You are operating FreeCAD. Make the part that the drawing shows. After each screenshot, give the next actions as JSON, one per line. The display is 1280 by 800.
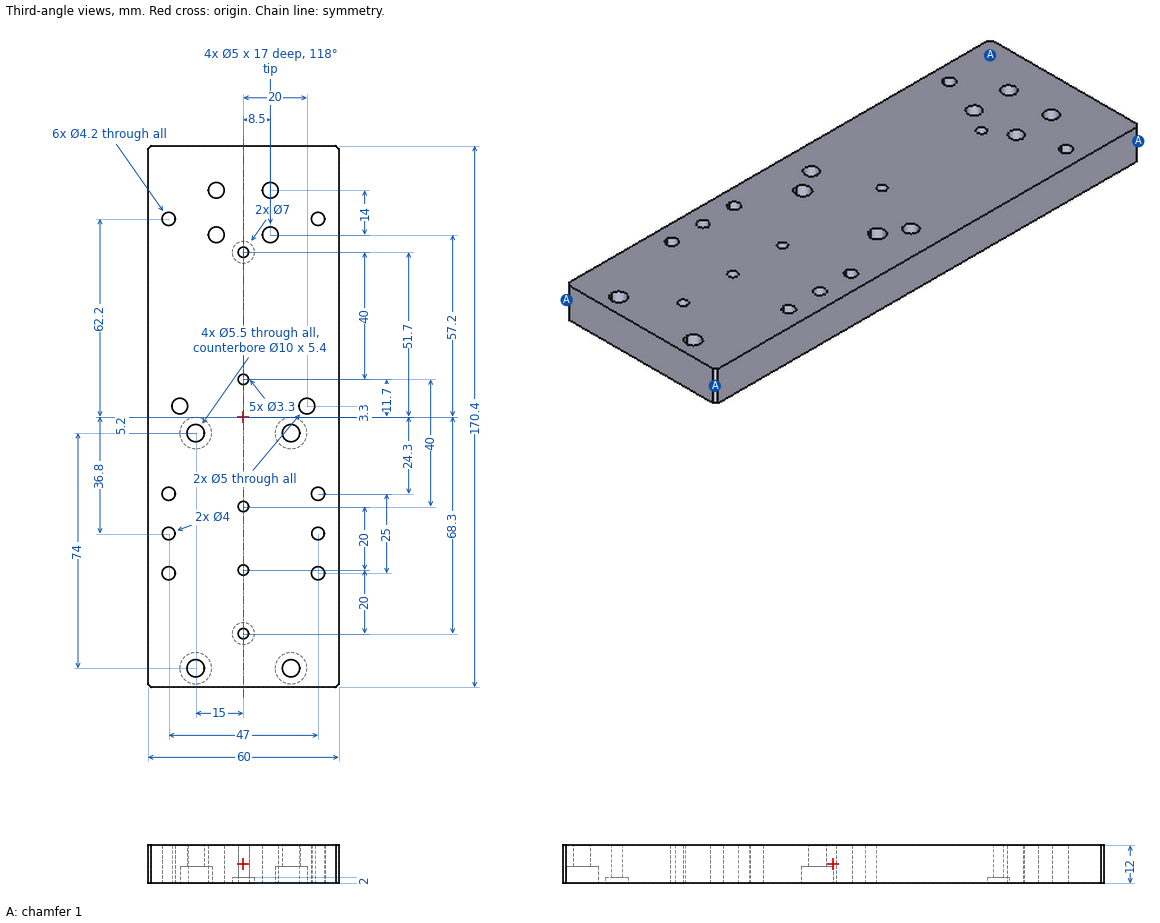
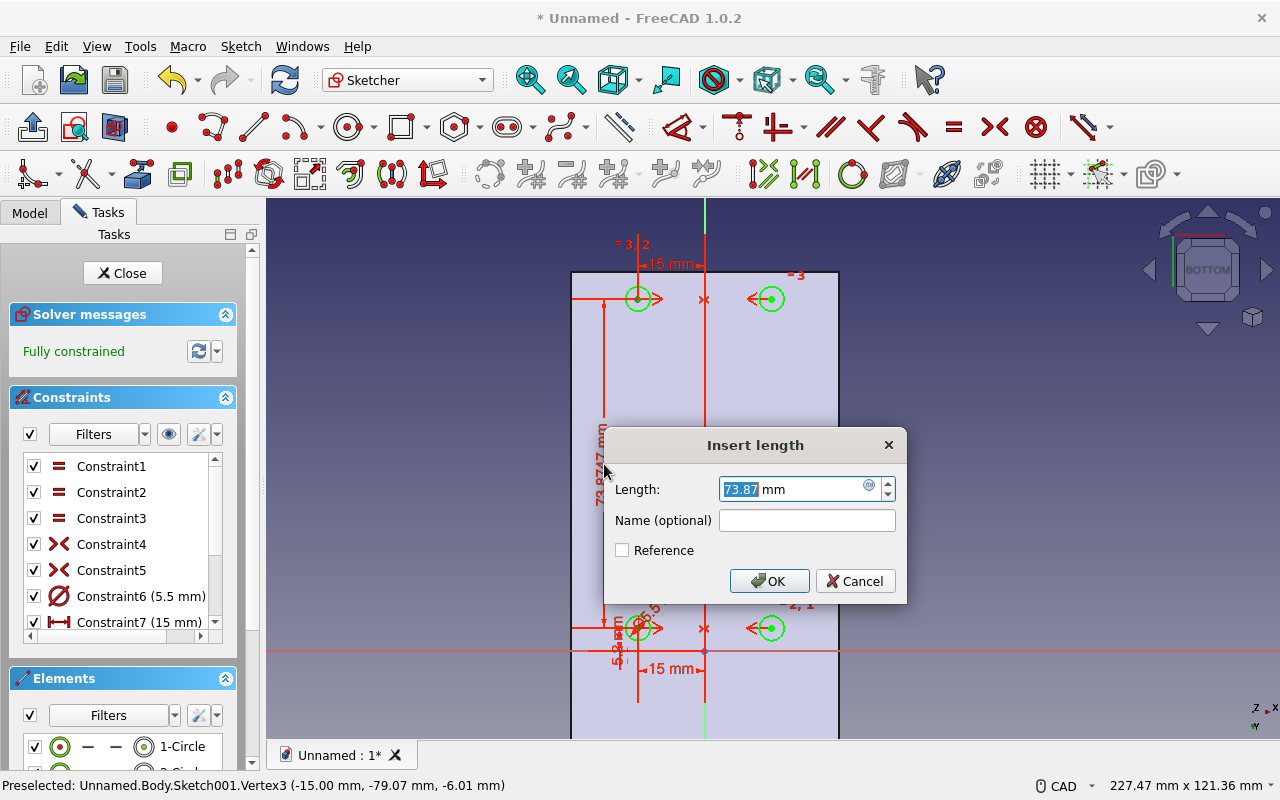
{"action": "type", "text": "74"}
{"action": "key", "text": "Return"}
{"action": "key", "text": "Escape"}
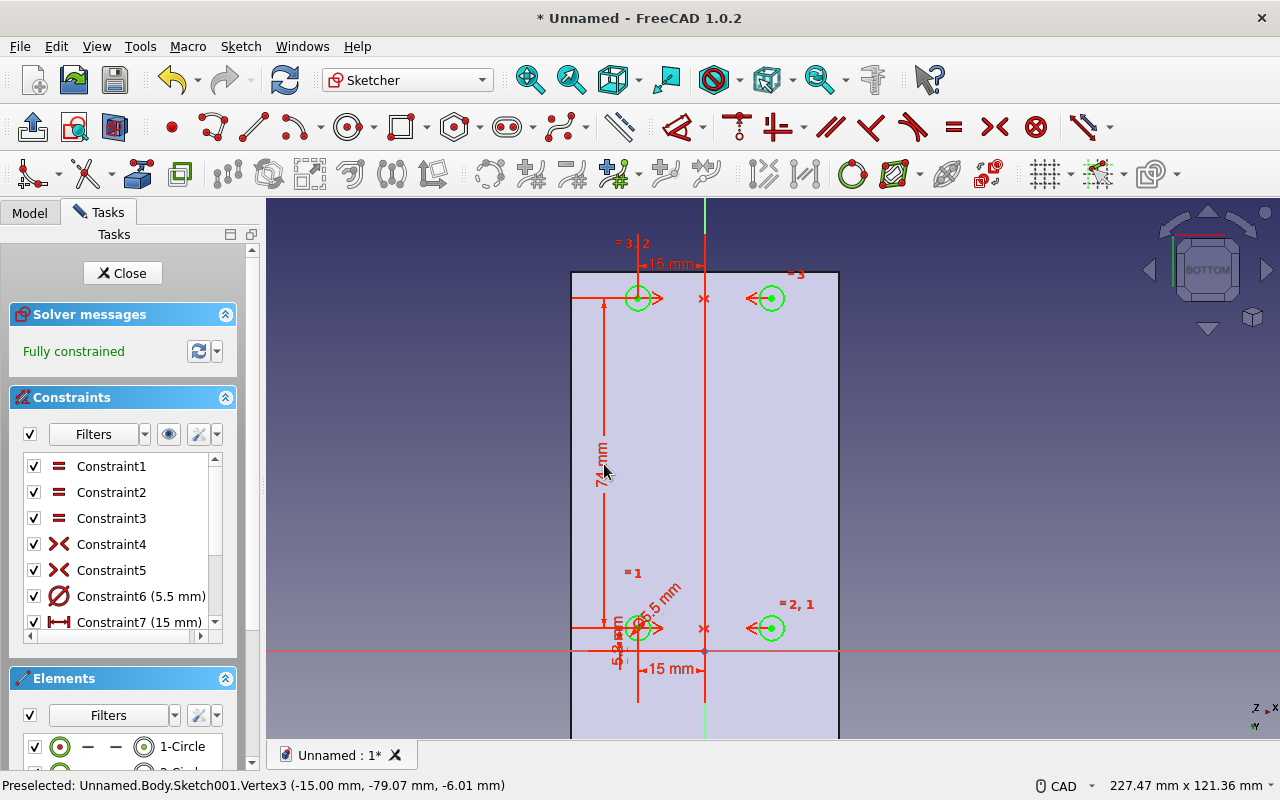
{"action": "left_click", "coordinate": [123, 273]}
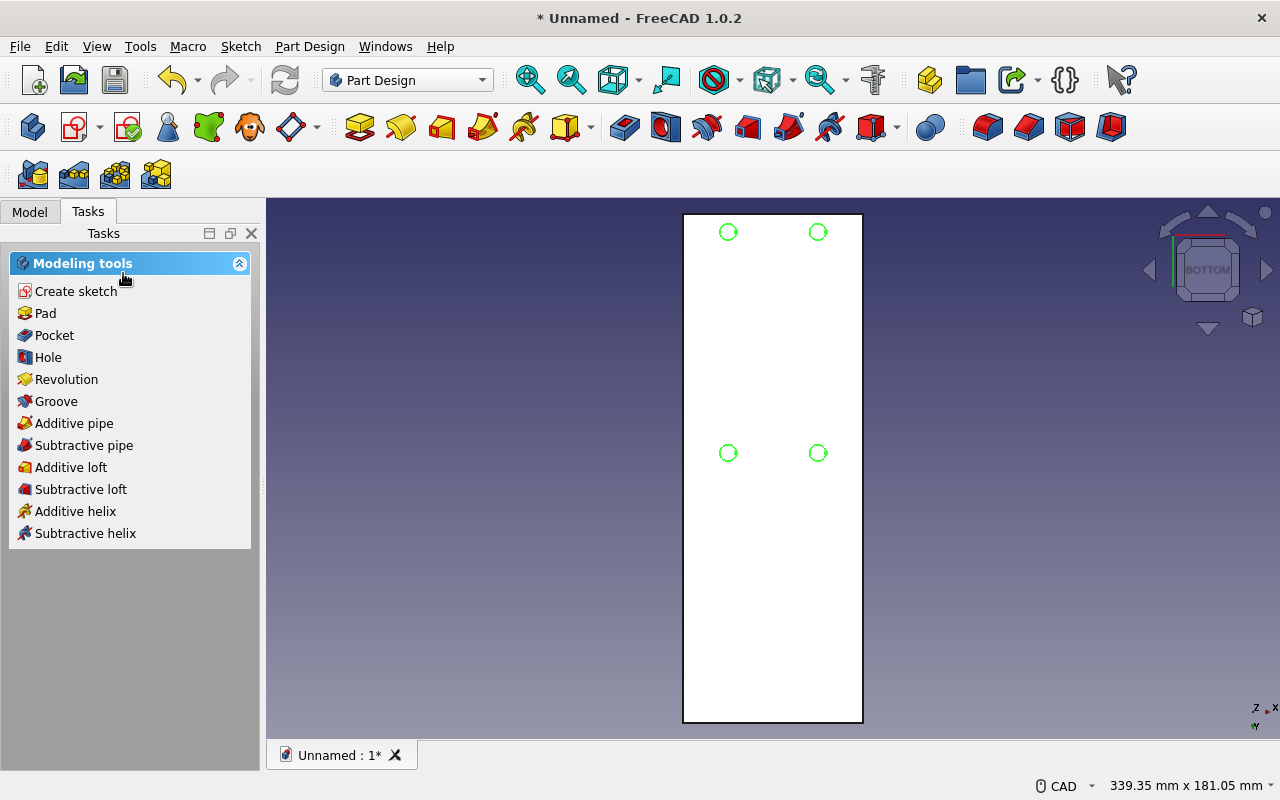
{"action": "left_click", "coordinate": [666, 128]}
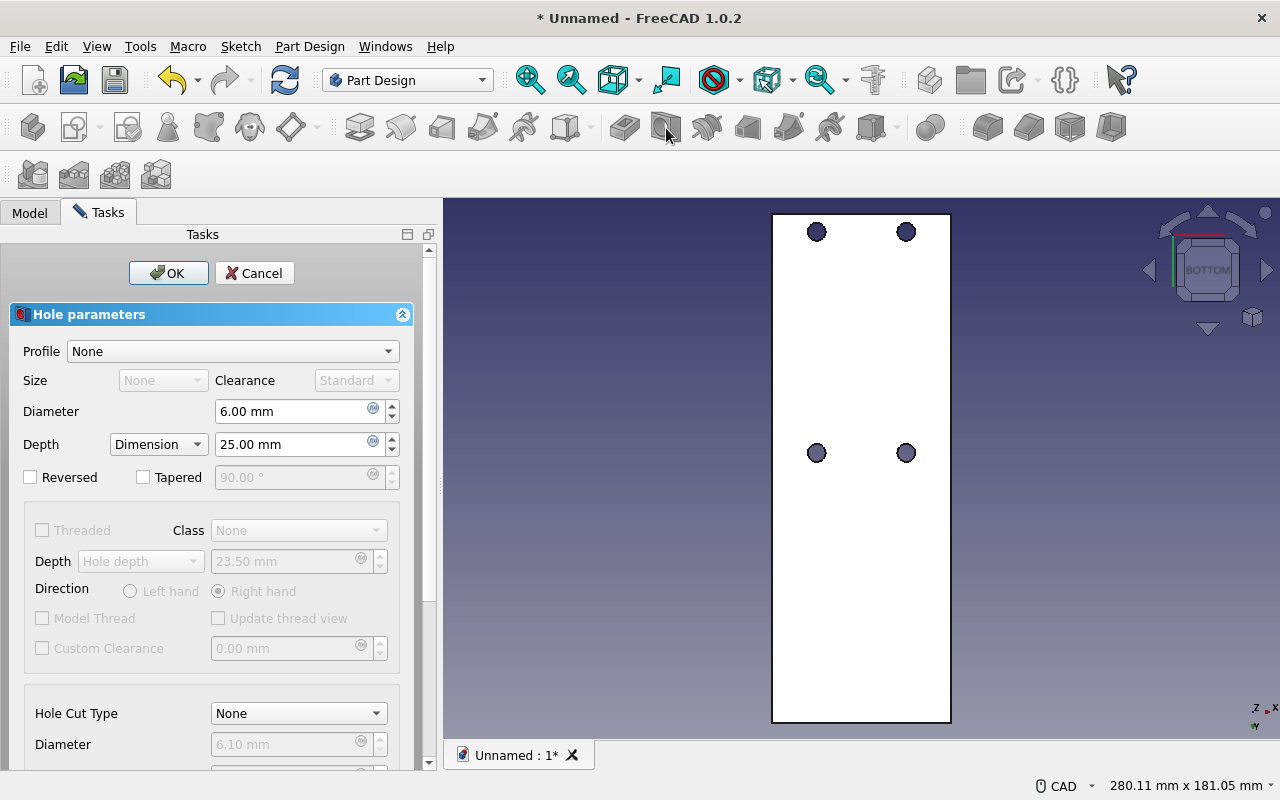
{"action": "triple_click", "coordinate": [300, 412]}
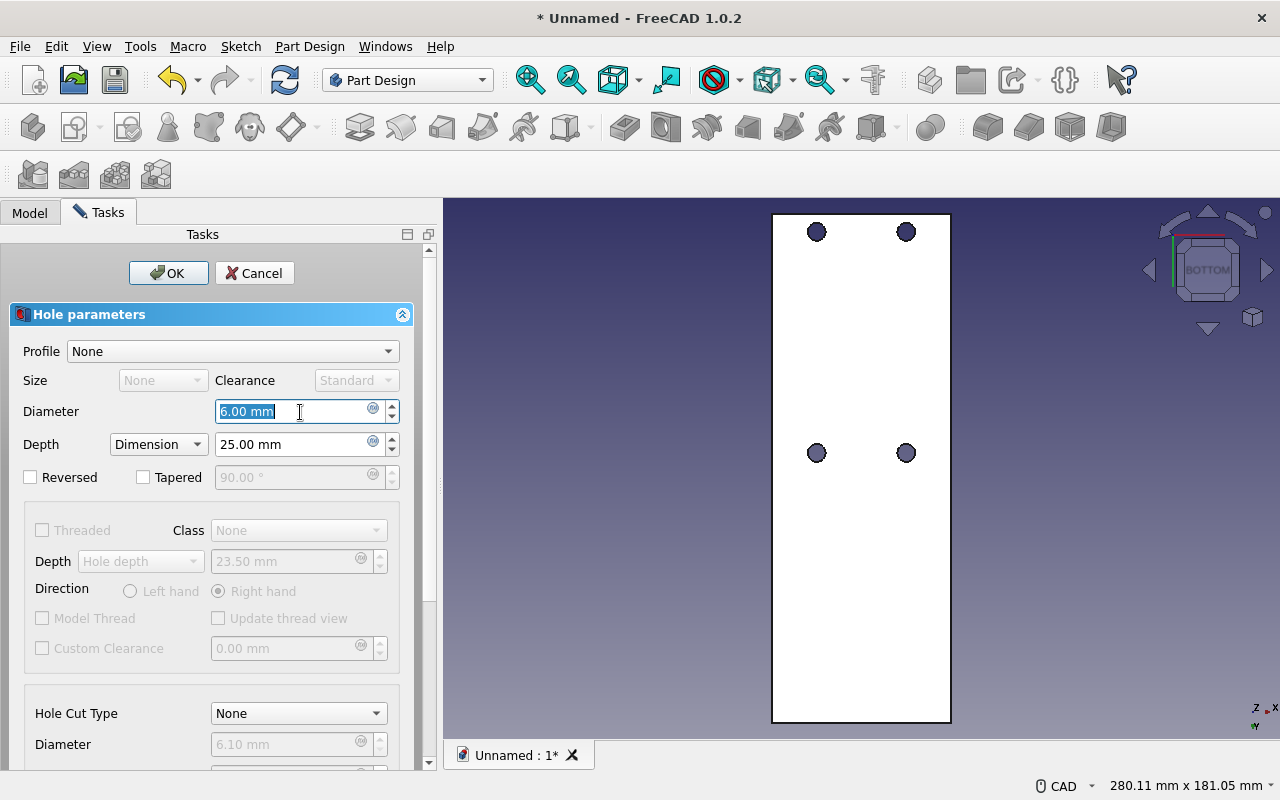
{"action": "type", "text": "5.5"}
{"action": "key", "text": "Tab"}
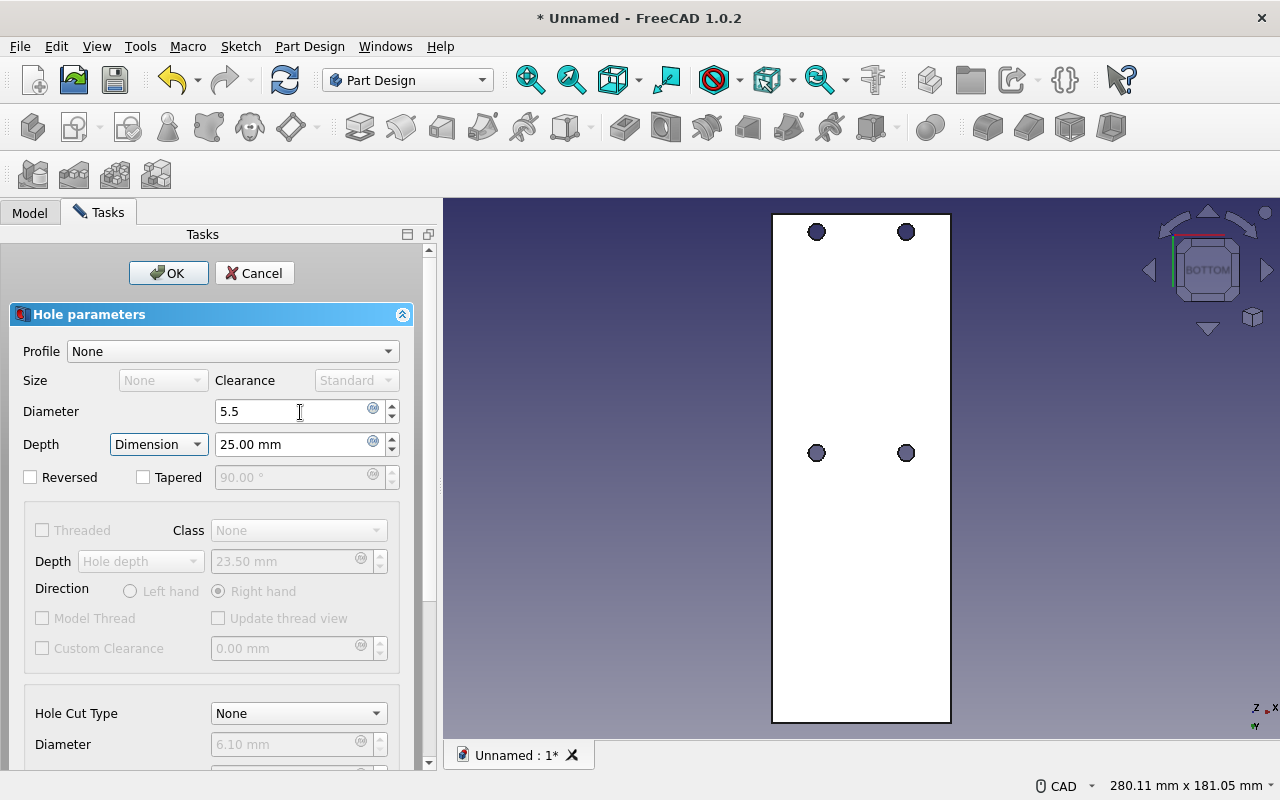
{"action": "left_click", "coordinate": [160, 444]}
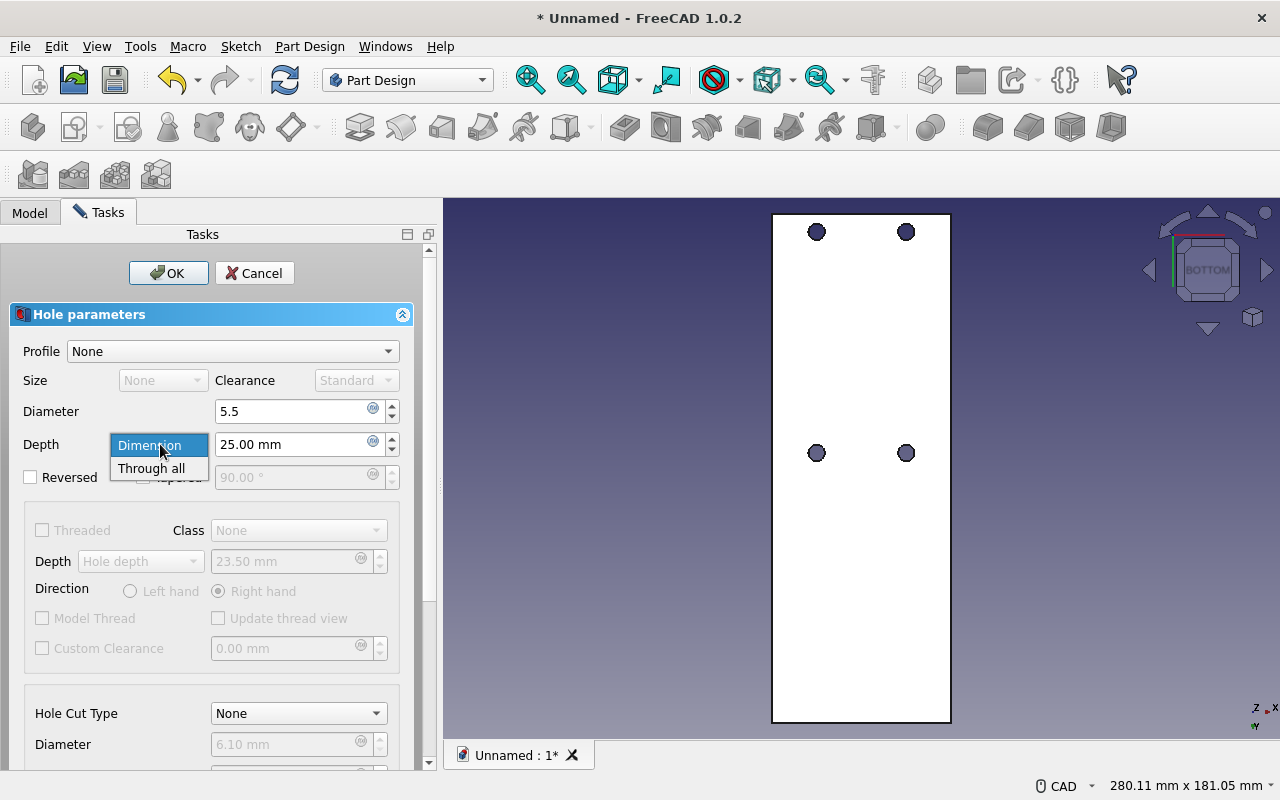
{"action": "left_click", "coordinate": [158, 468]}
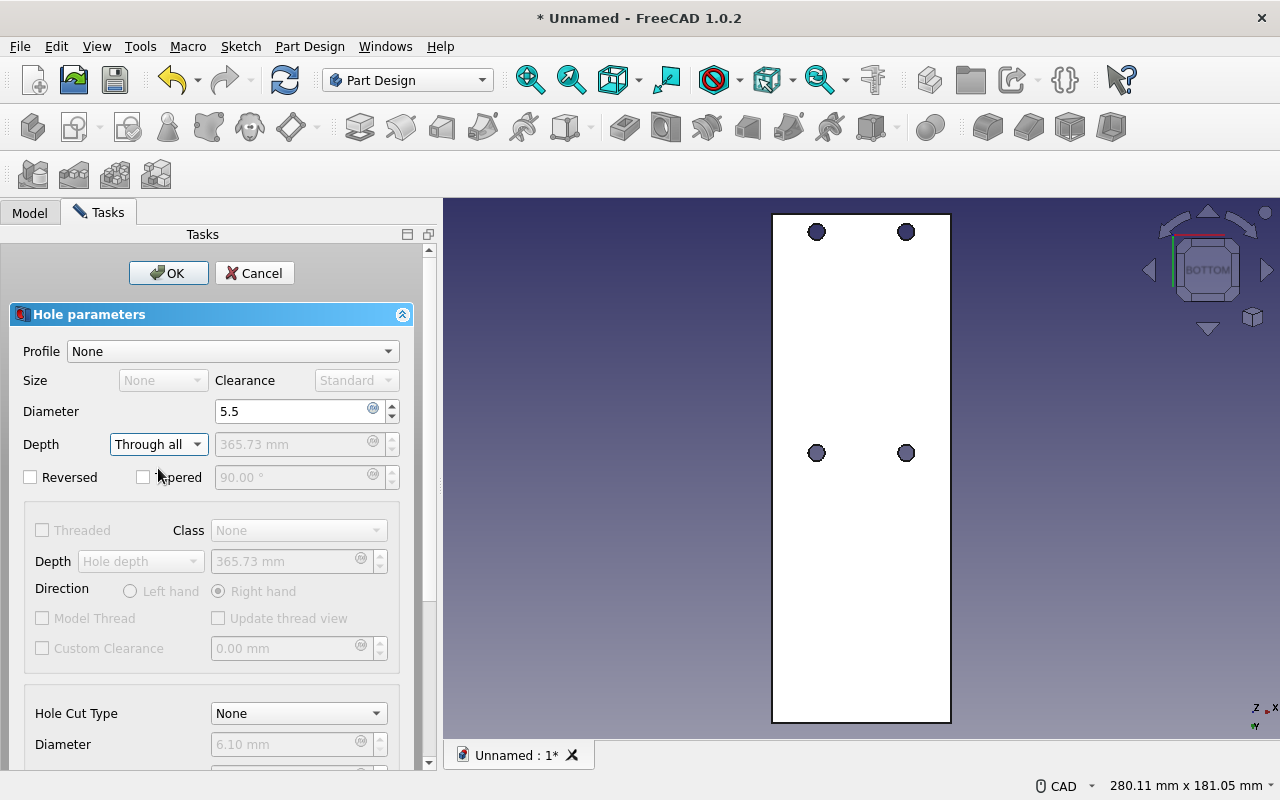
{"action": "left_click", "coordinate": [300, 714]}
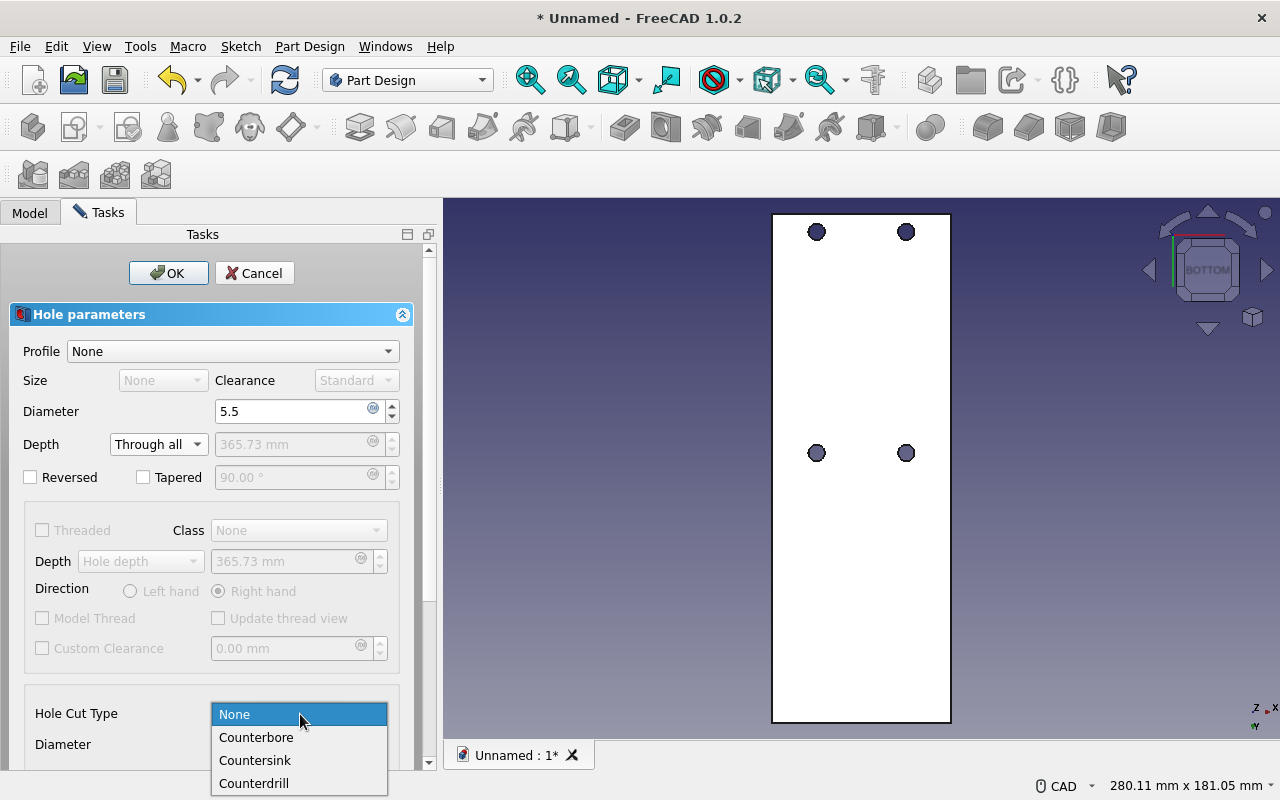
{"action": "left_click", "coordinate": [298, 738]}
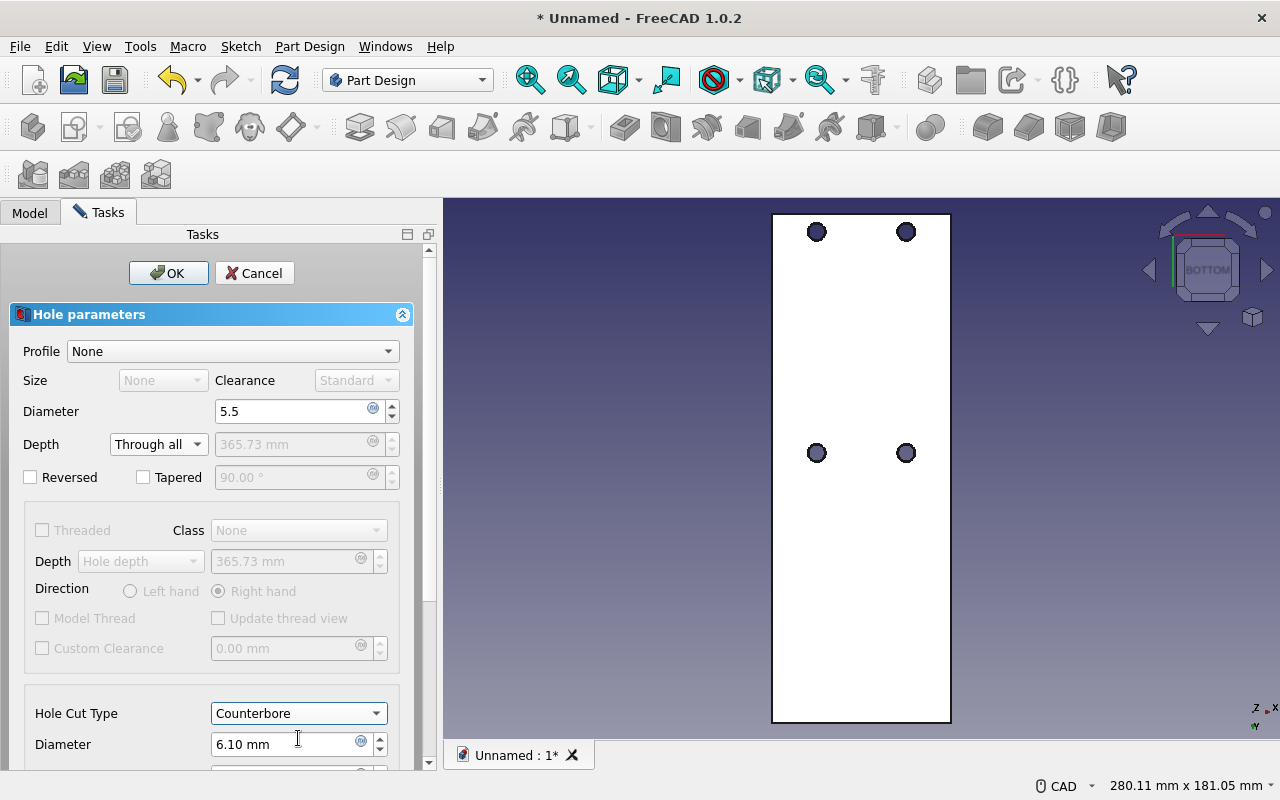
{"action": "triple_click", "coordinate": [292, 744]}